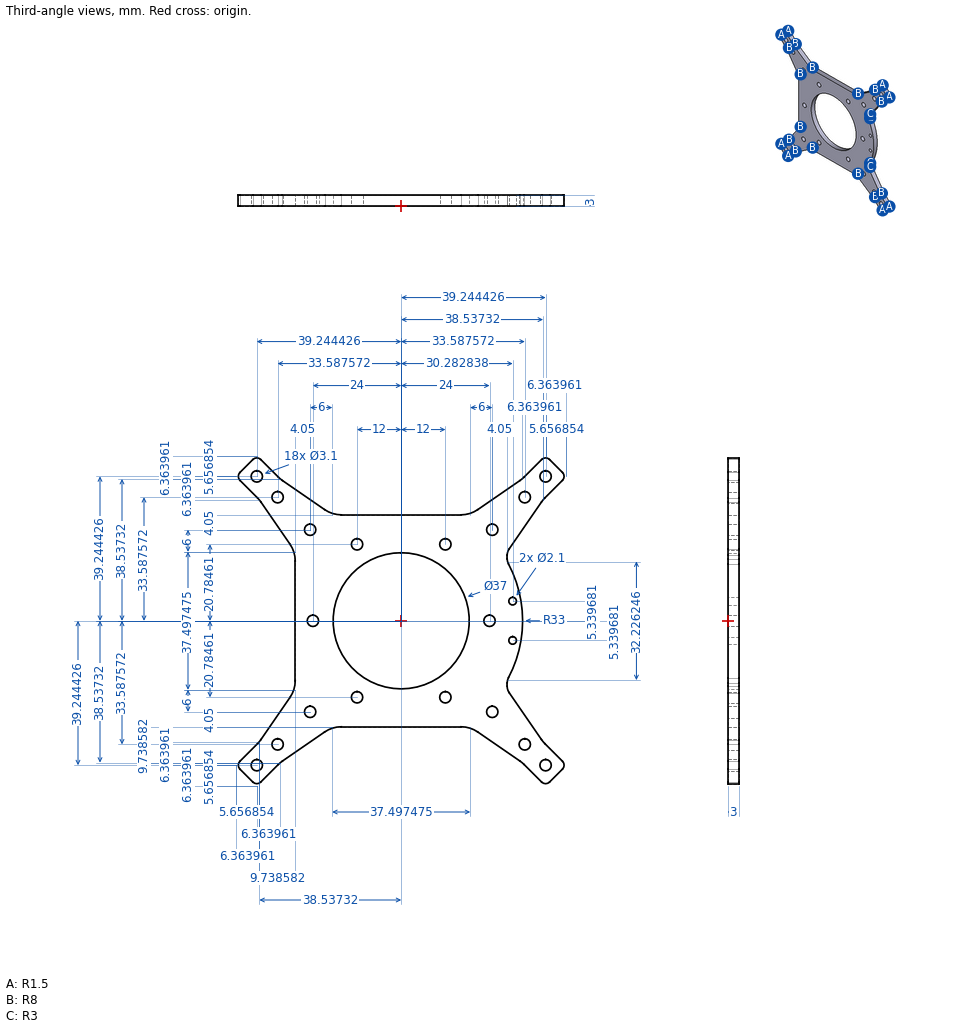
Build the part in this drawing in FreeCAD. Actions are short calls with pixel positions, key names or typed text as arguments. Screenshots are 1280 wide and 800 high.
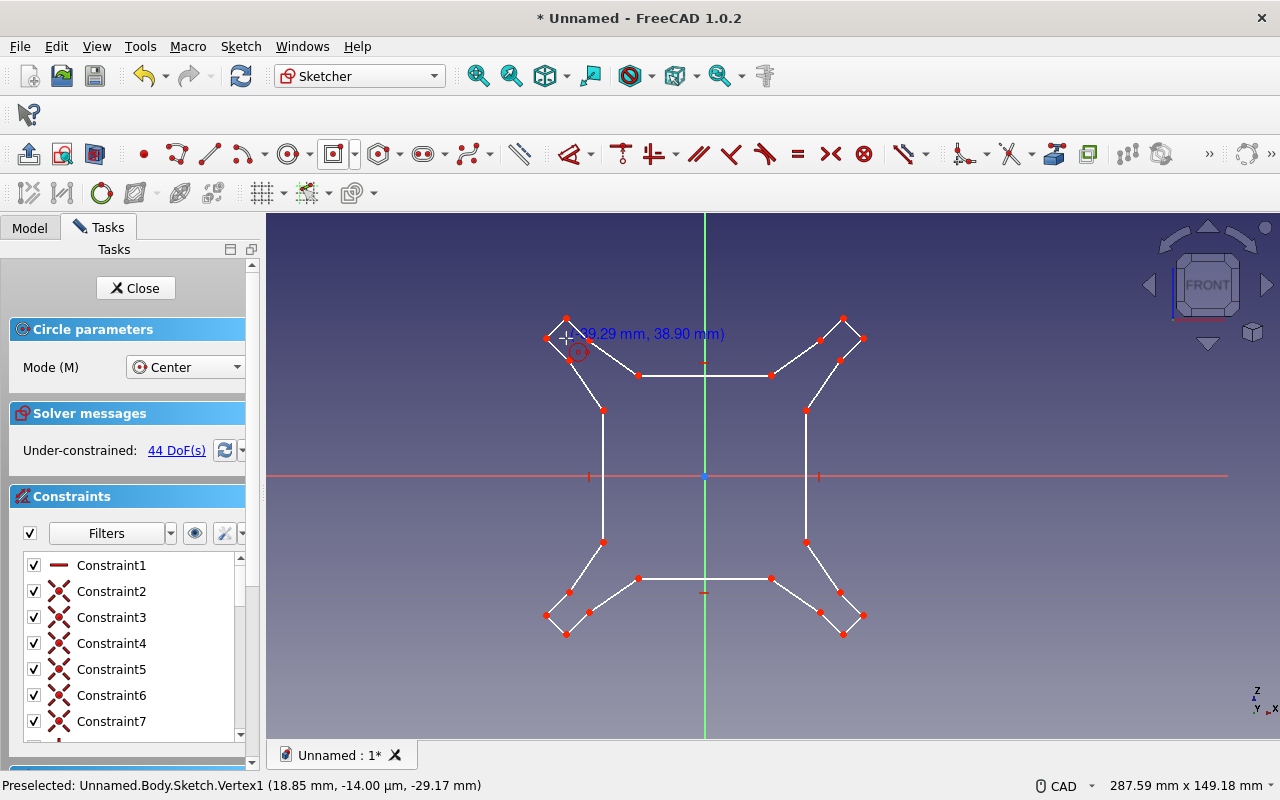
click(566, 338)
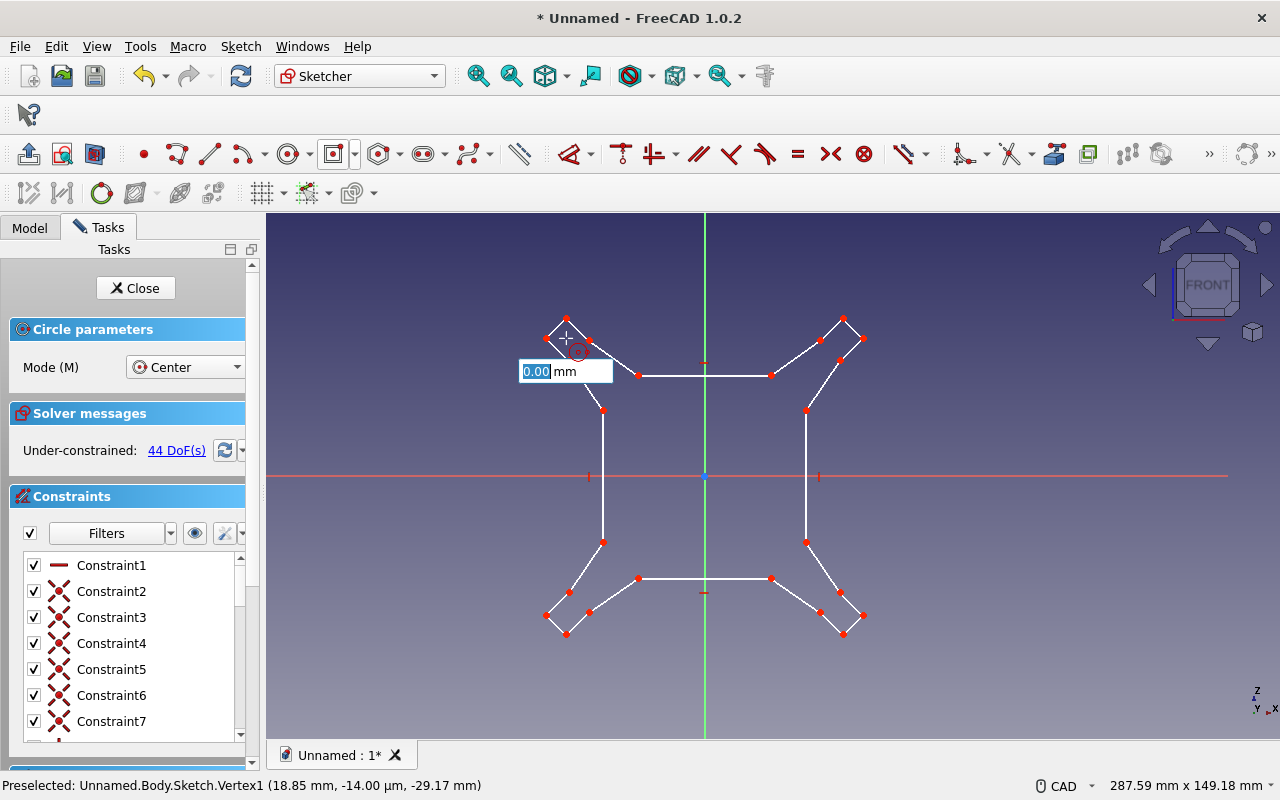
scroll(570, 342, up, 6)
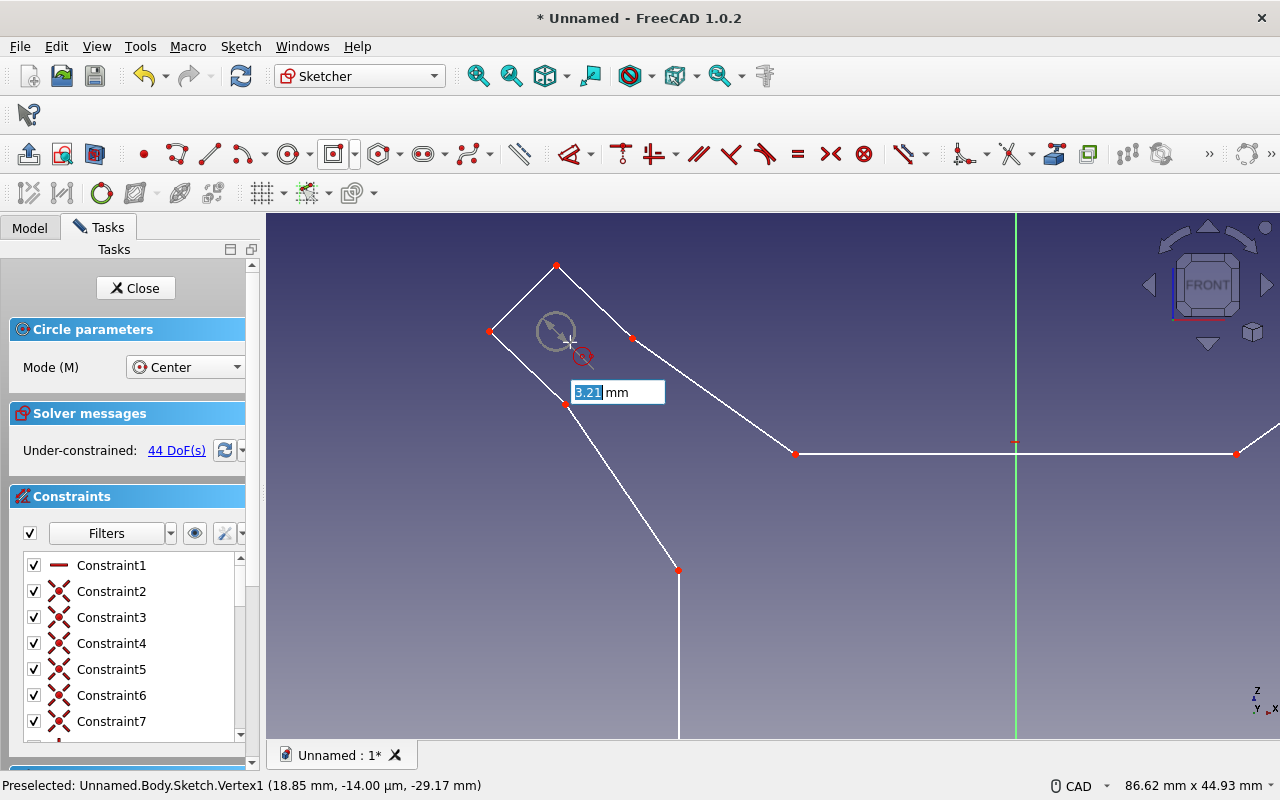
click(569, 340)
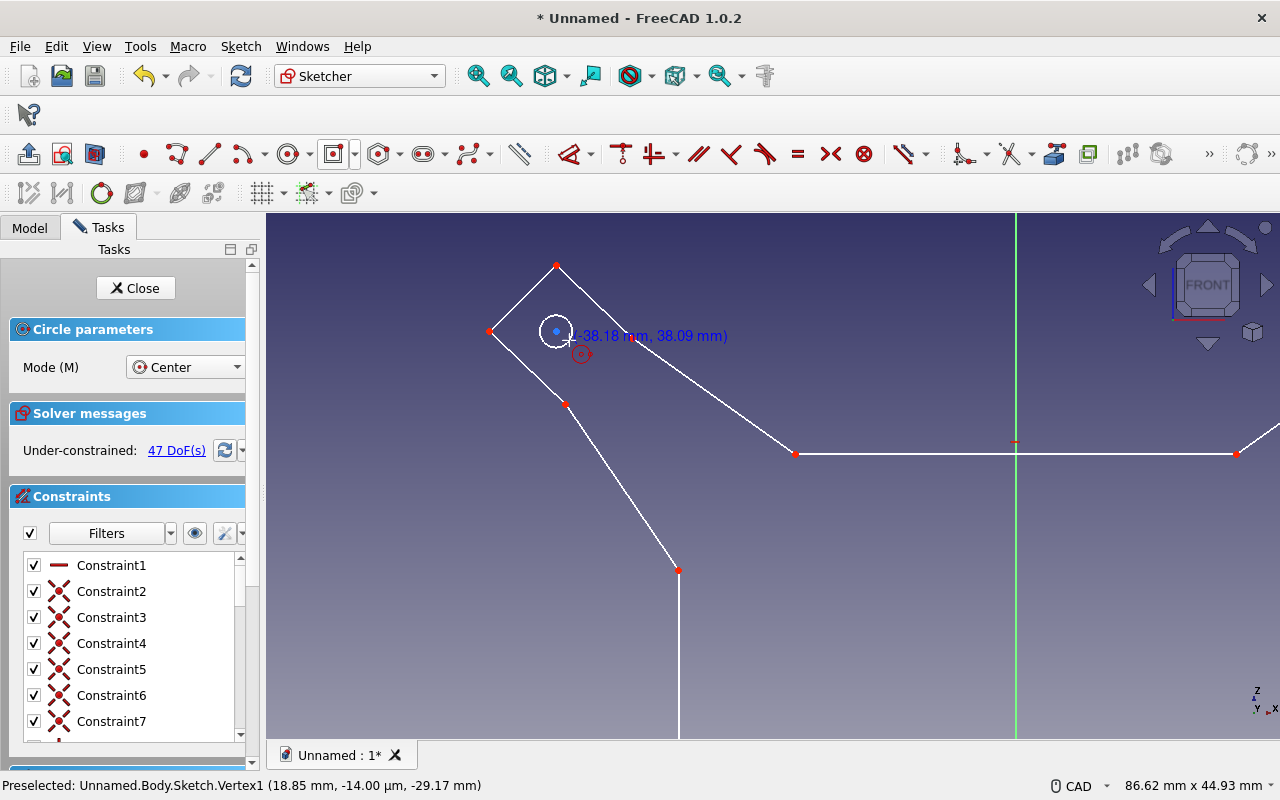
scroll(623, 394, up, 2)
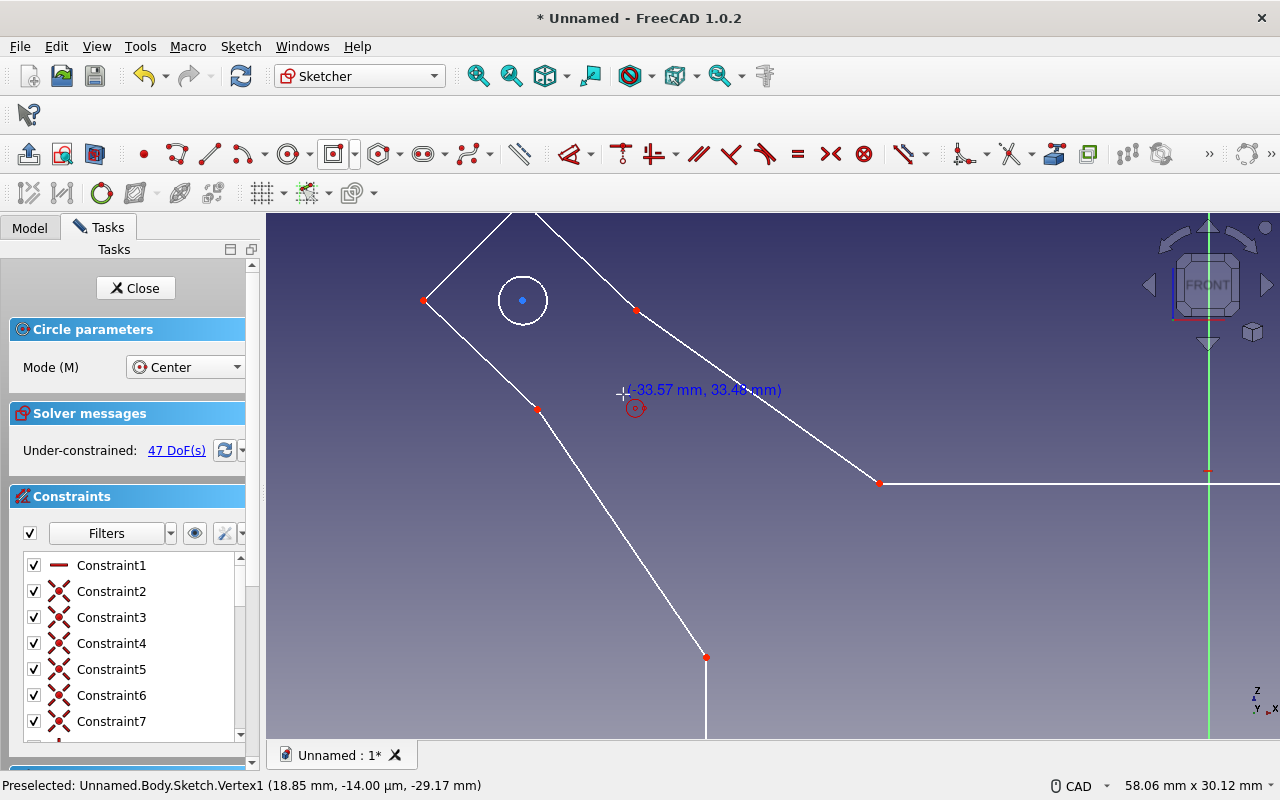
scroll(577, 349, down, 8)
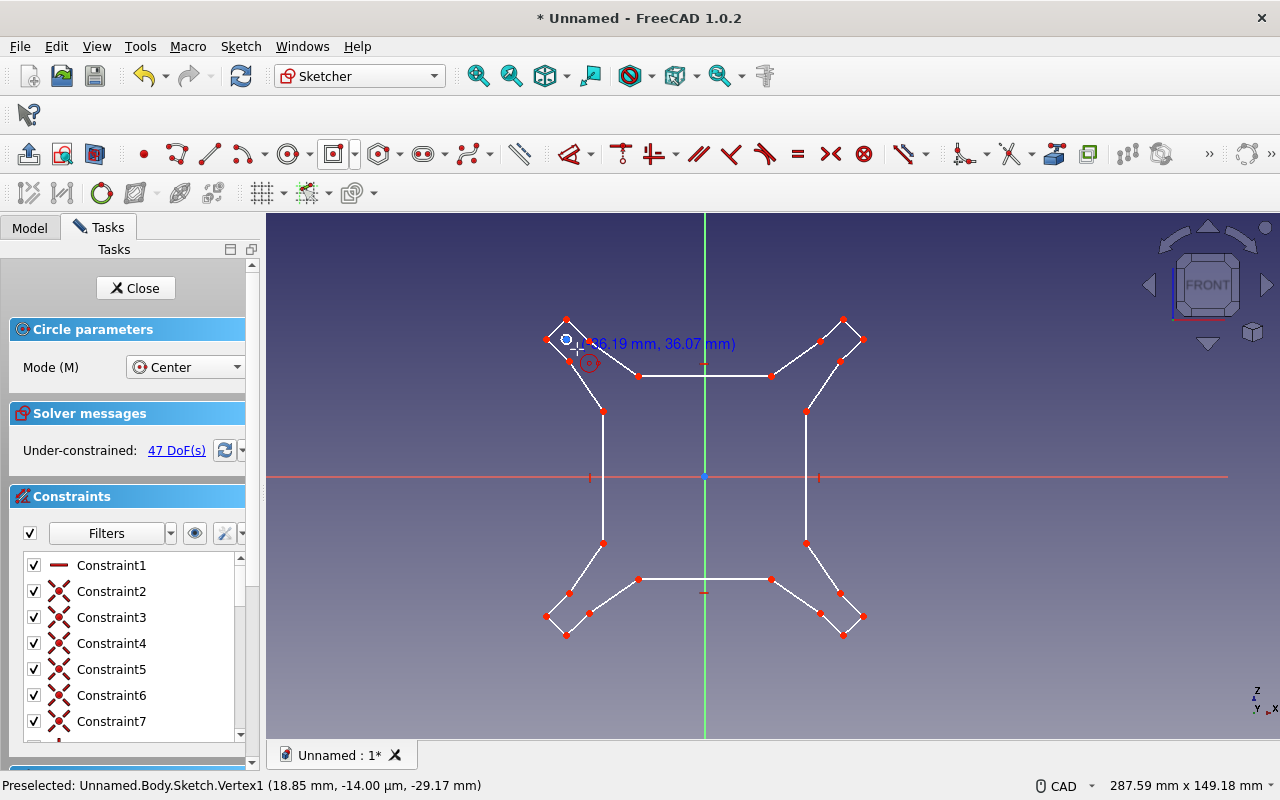
click(586, 358)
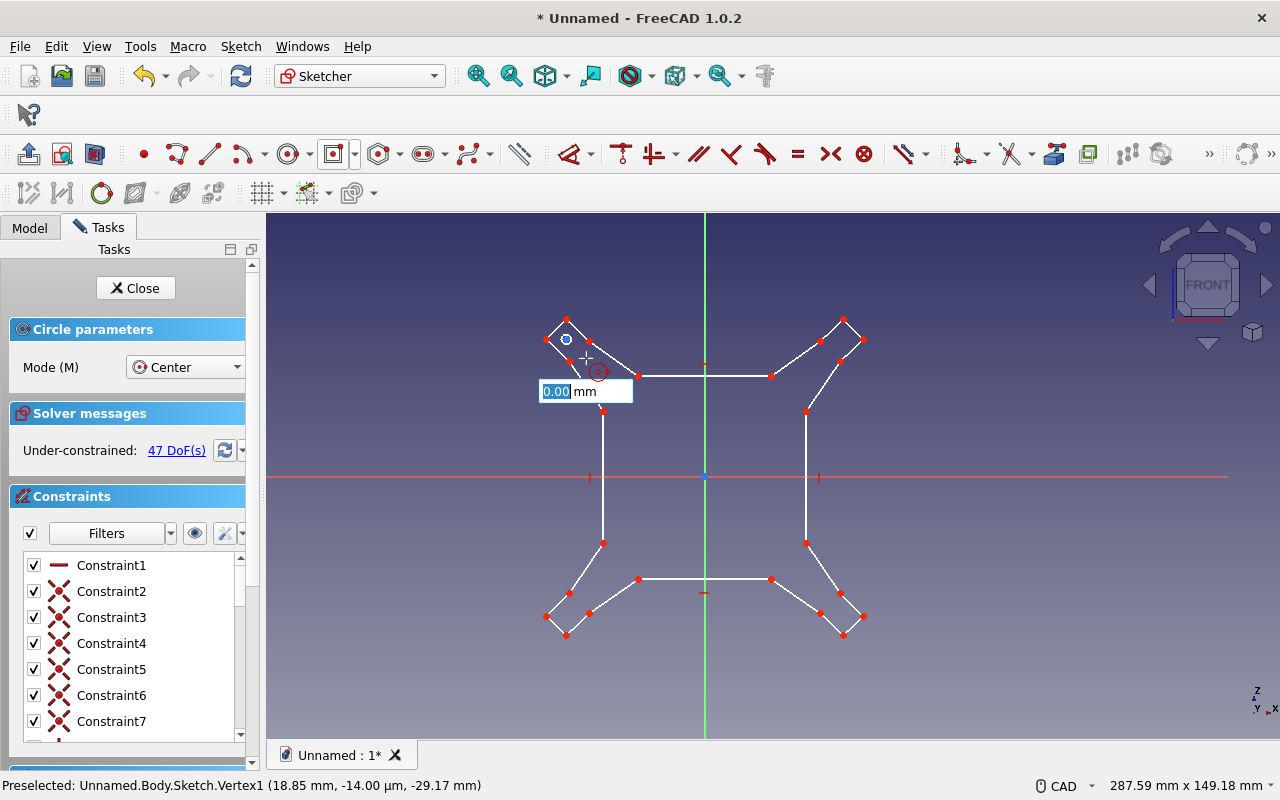
scroll(583, 354, up, 6)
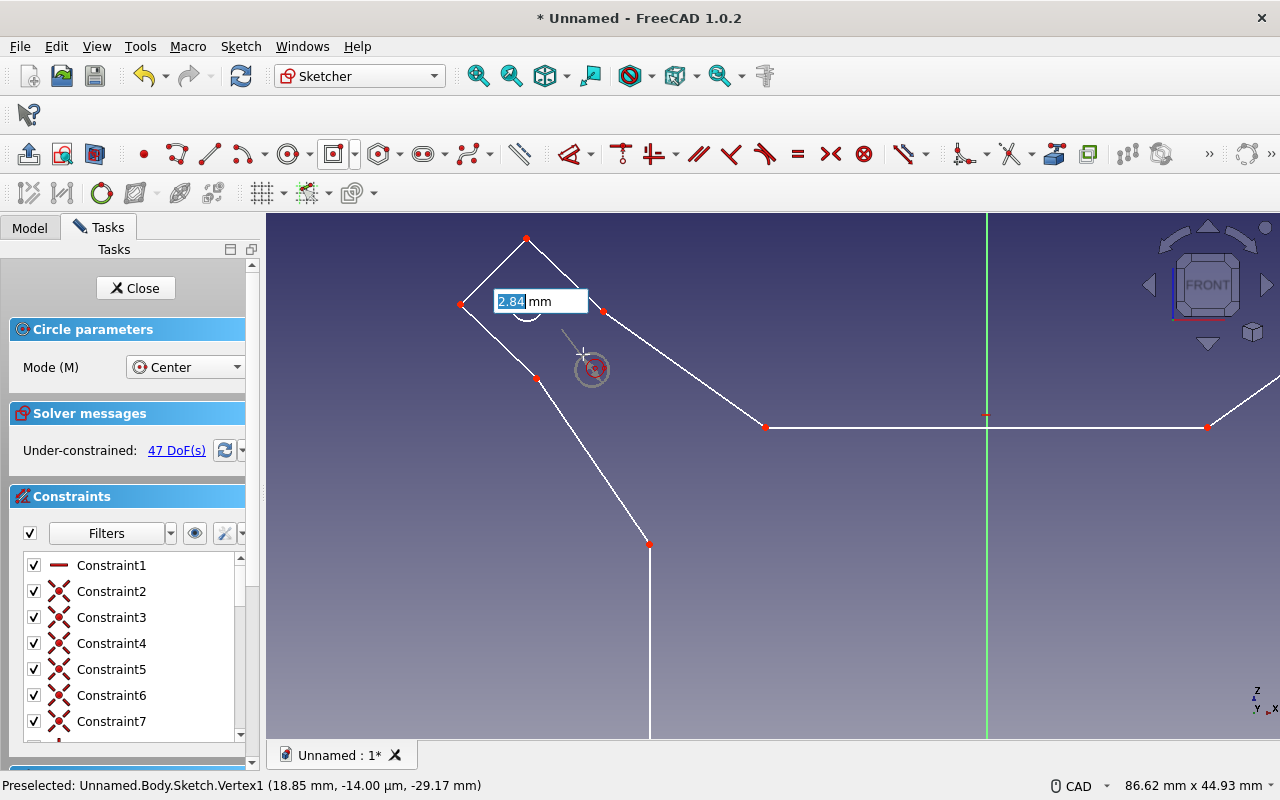
click(581, 354)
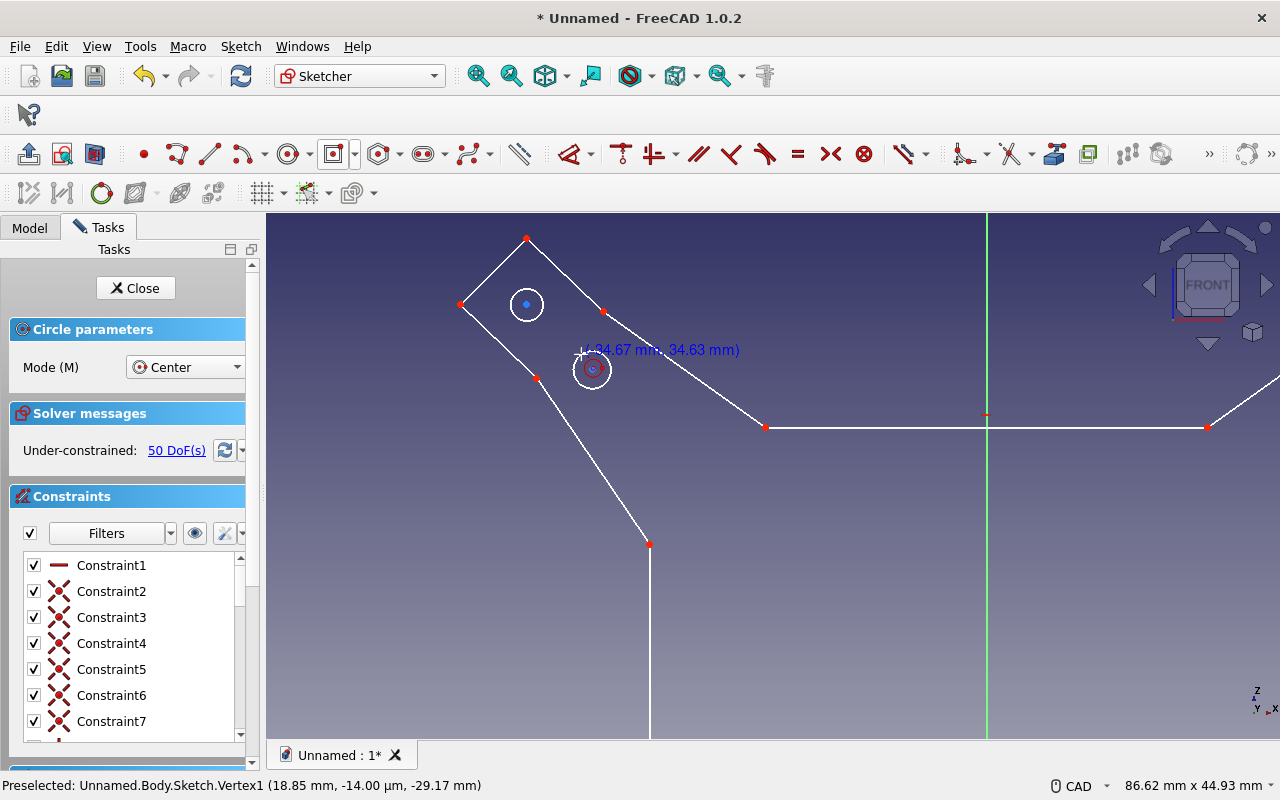
scroll(697, 471, up, 2)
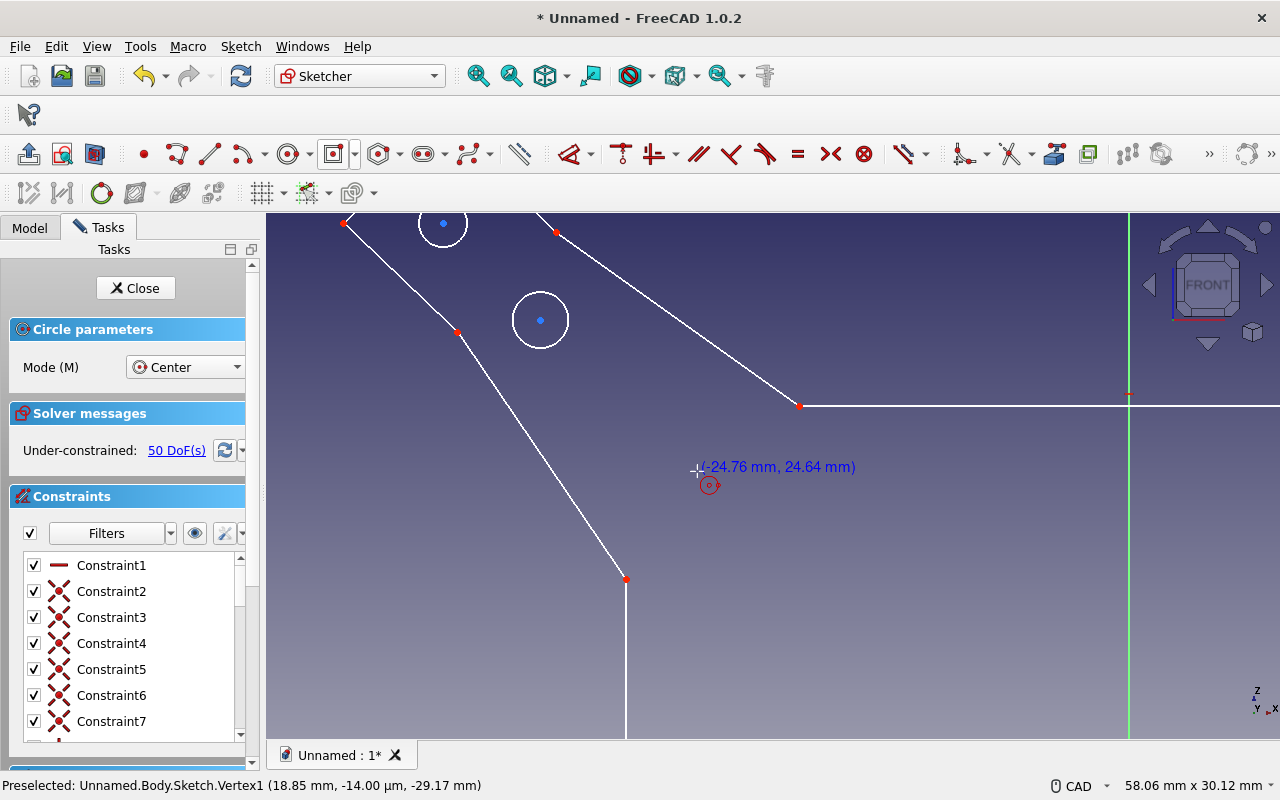
scroll(597, 368, down, 8)